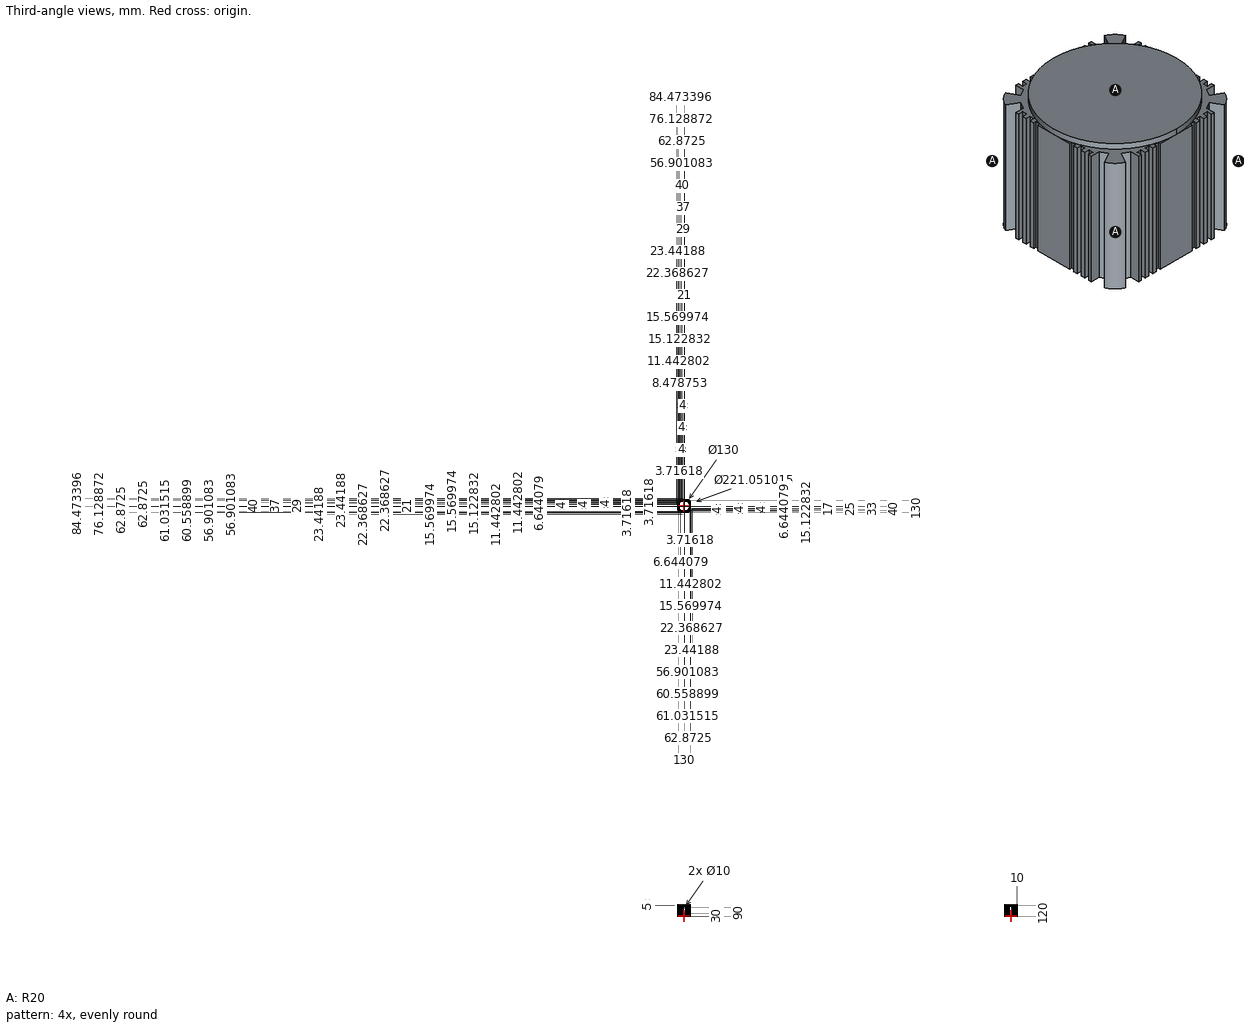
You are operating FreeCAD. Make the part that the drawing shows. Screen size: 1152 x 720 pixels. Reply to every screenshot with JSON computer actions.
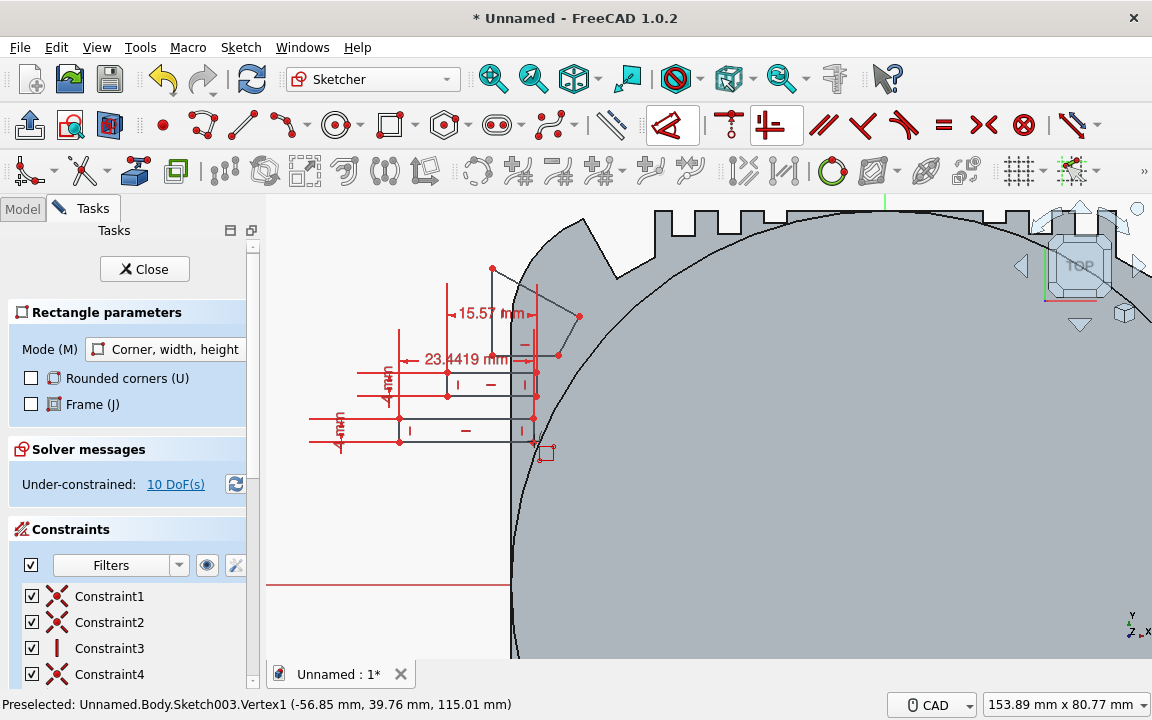
{"action": "left_click", "coordinate": [395, 464]}
{"action": "mouse_move", "coordinate": [523, 487]}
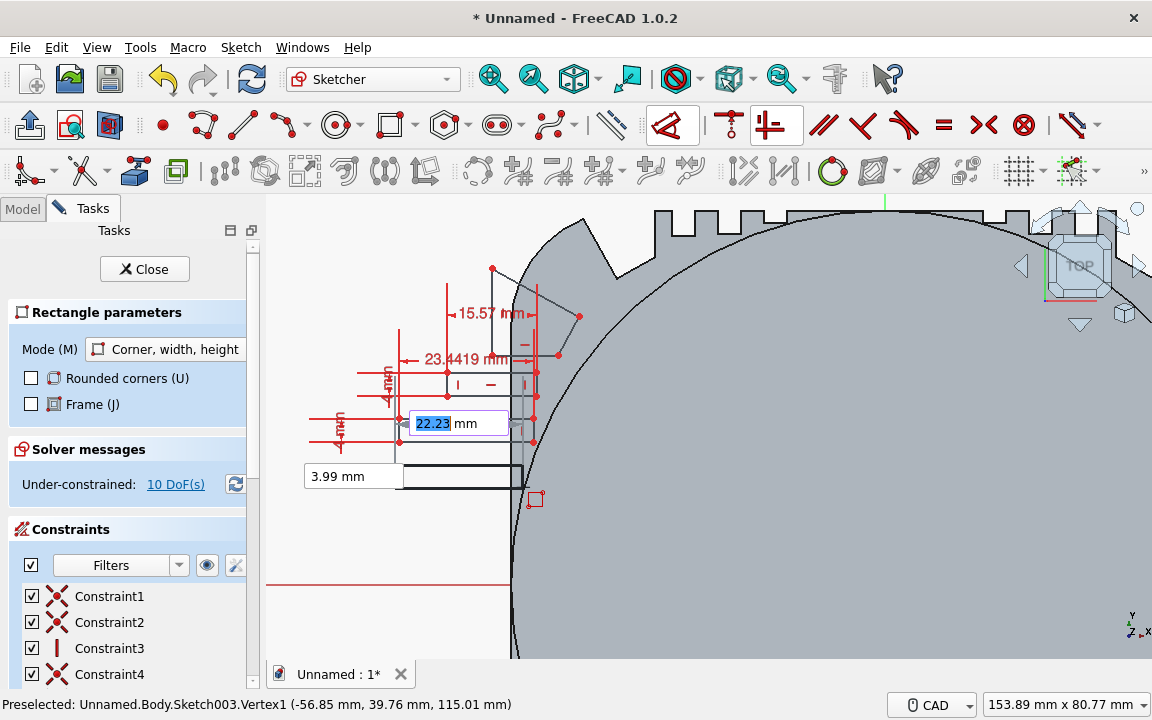
{"action": "type", "text": "22.368627"}
{"action": "key", "text": "Tab"}
{"action": "type", "text": "4"}
{"action": "key", "text": "Return"}
{"action": "key", "text": "Escape"}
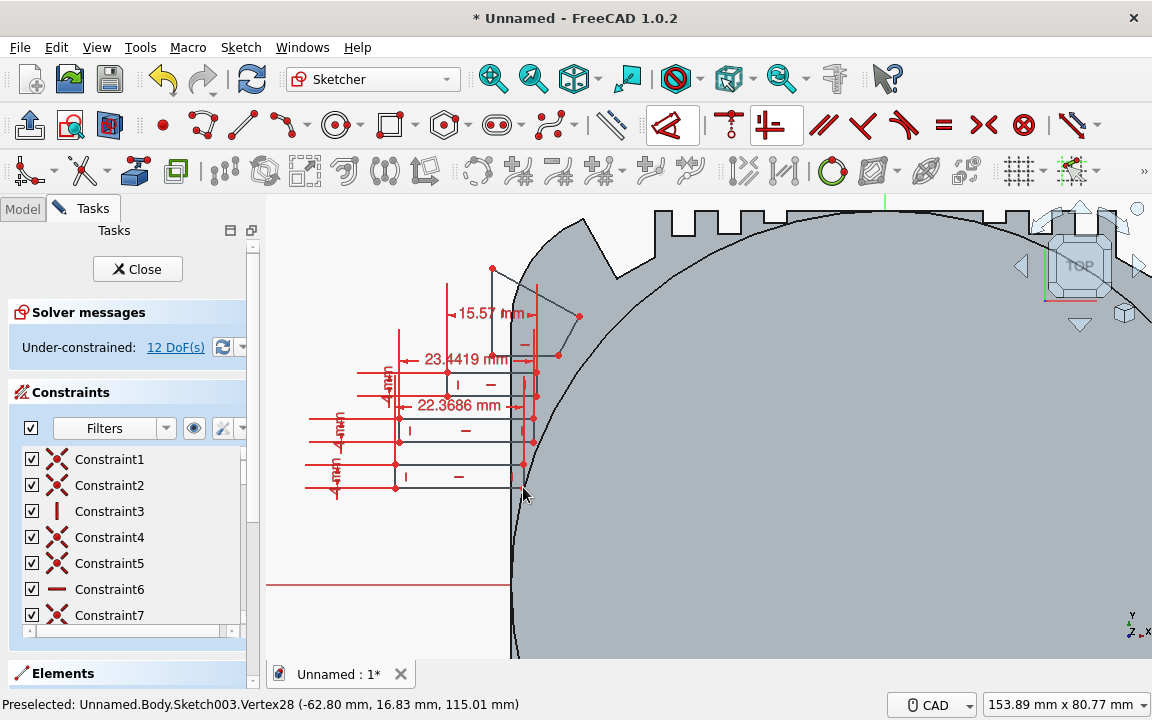
{"action": "left_click", "coordinate": [558, 356]}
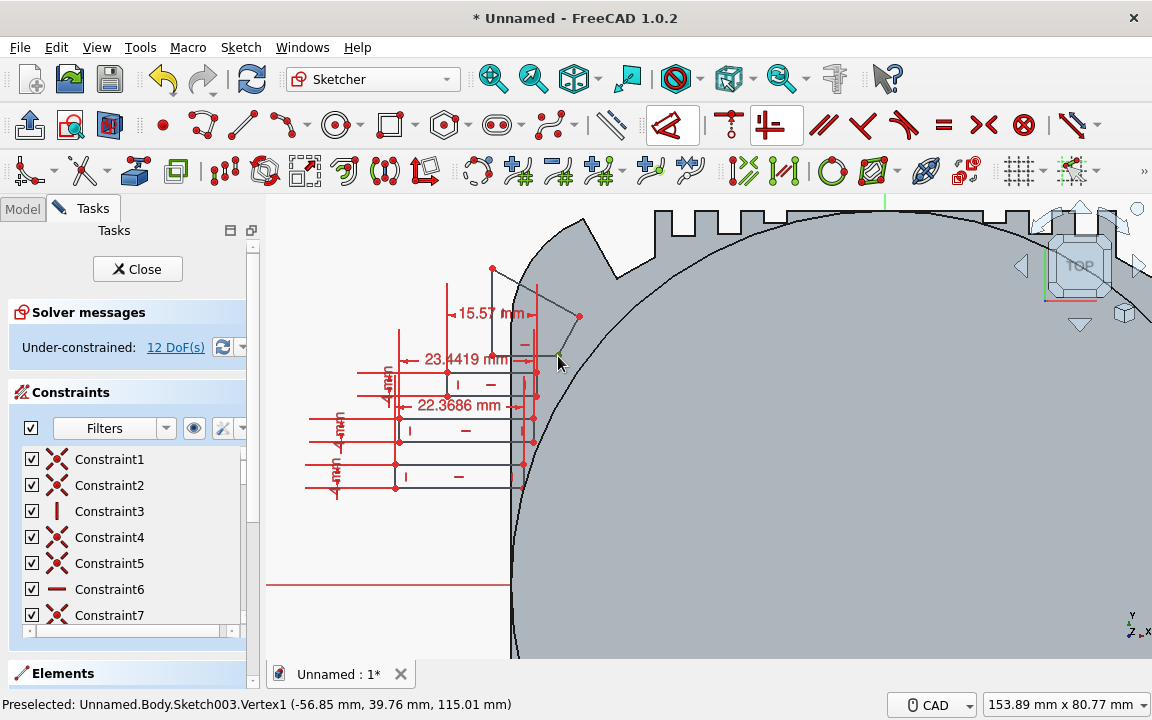
{"action": "key", "text": "i"}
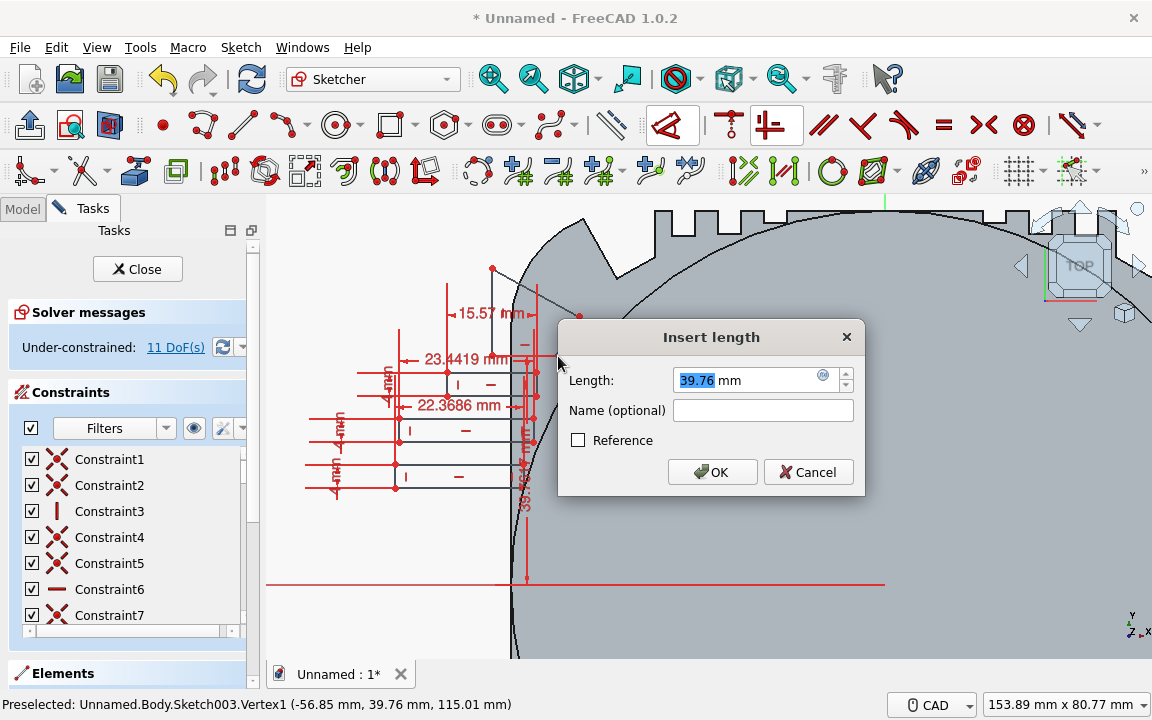
{"action": "type", "text": "40"}
{"action": "key", "text": "Return"}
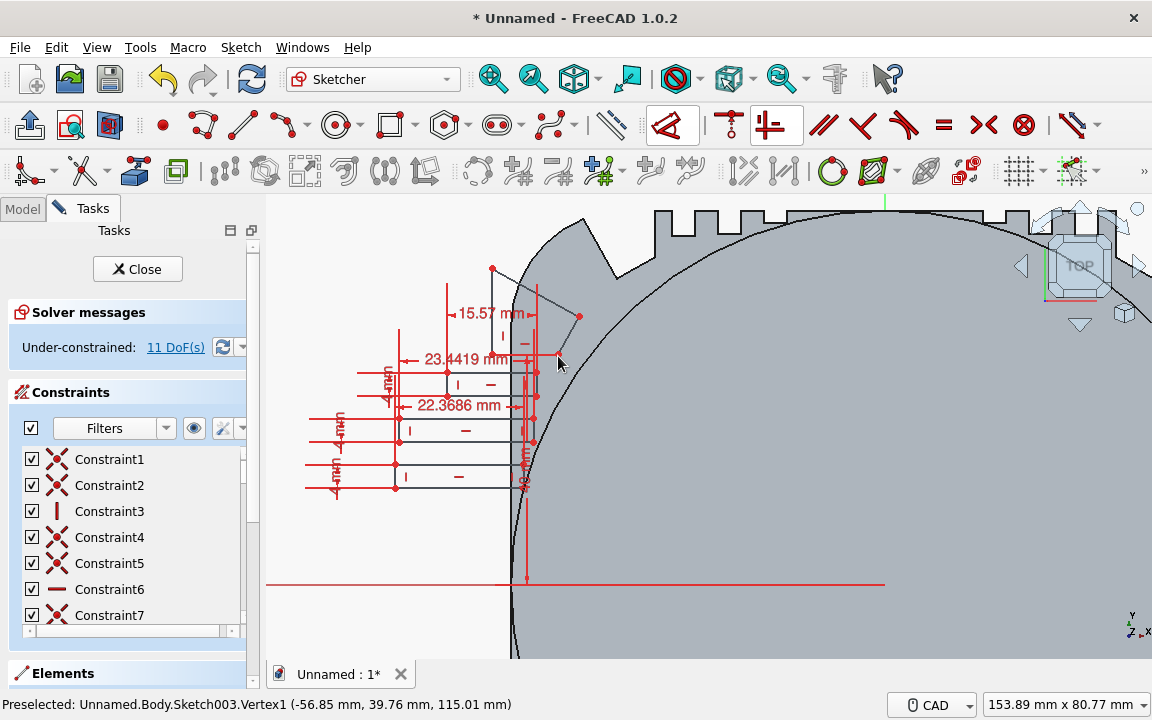
{"action": "left_click", "coordinate": [447, 373]}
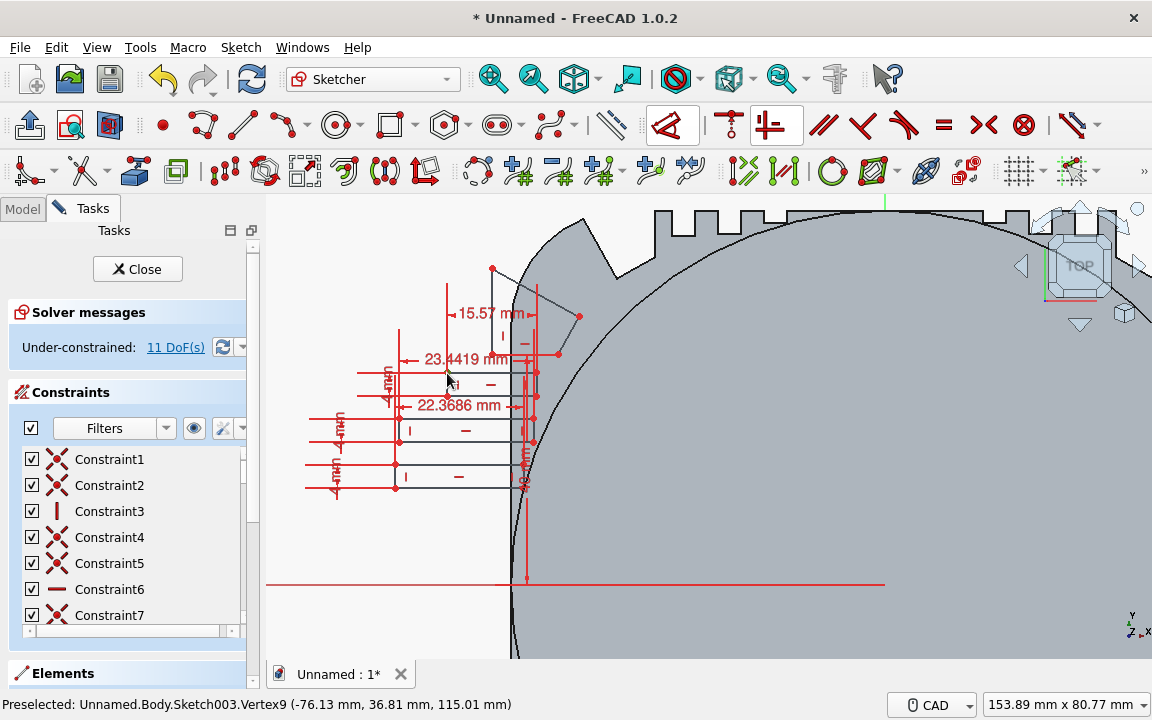
{"action": "left_click", "coordinate": [694, 126]}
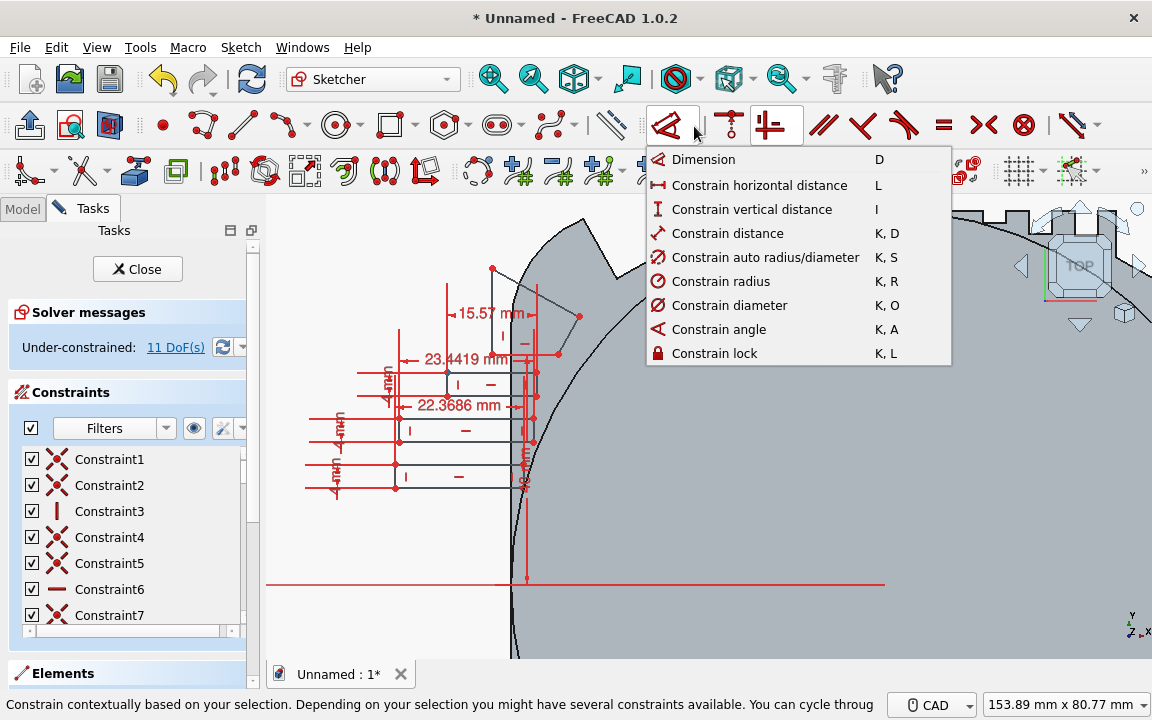
{"action": "left_click", "coordinate": [799, 209]}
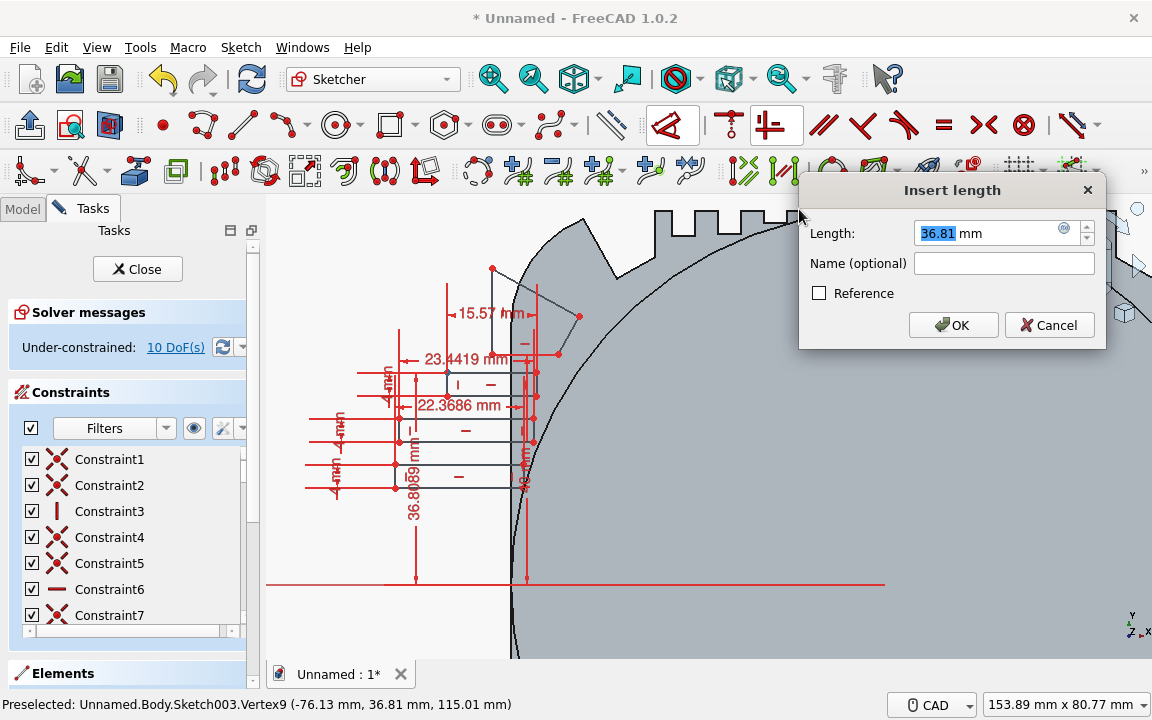
{"action": "type", "text": "37"}
{"action": "key", "text": "Return"}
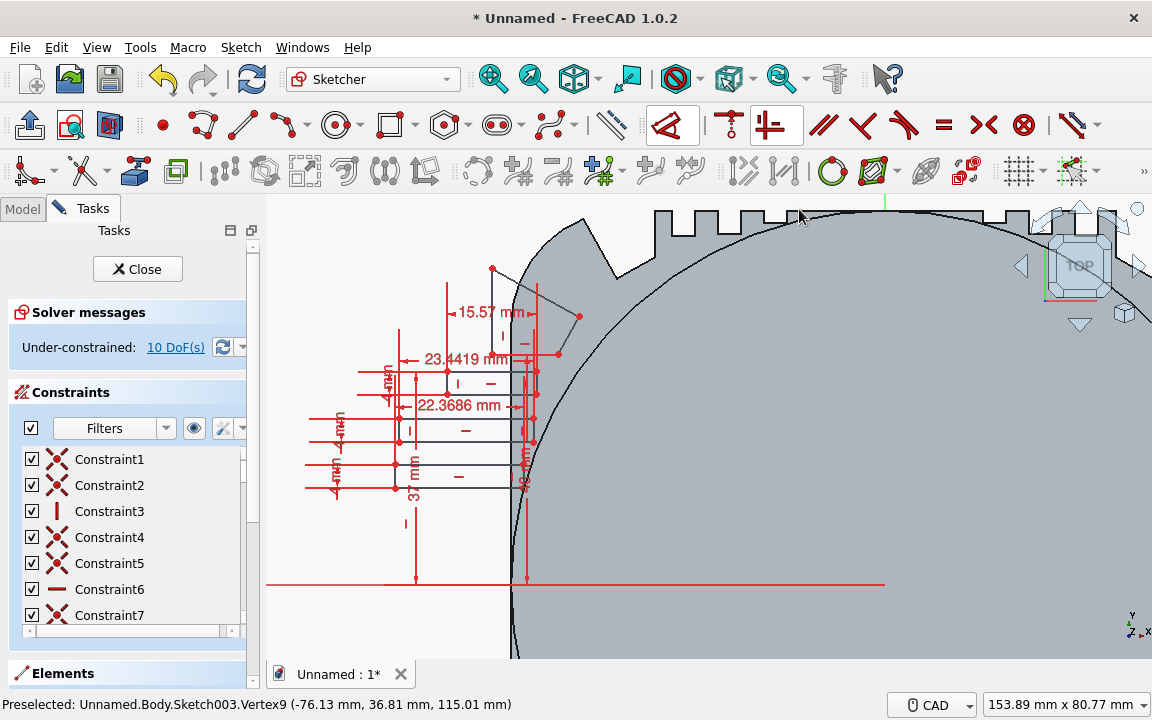
{"action": "left_click", "coordinate": [399, 419]}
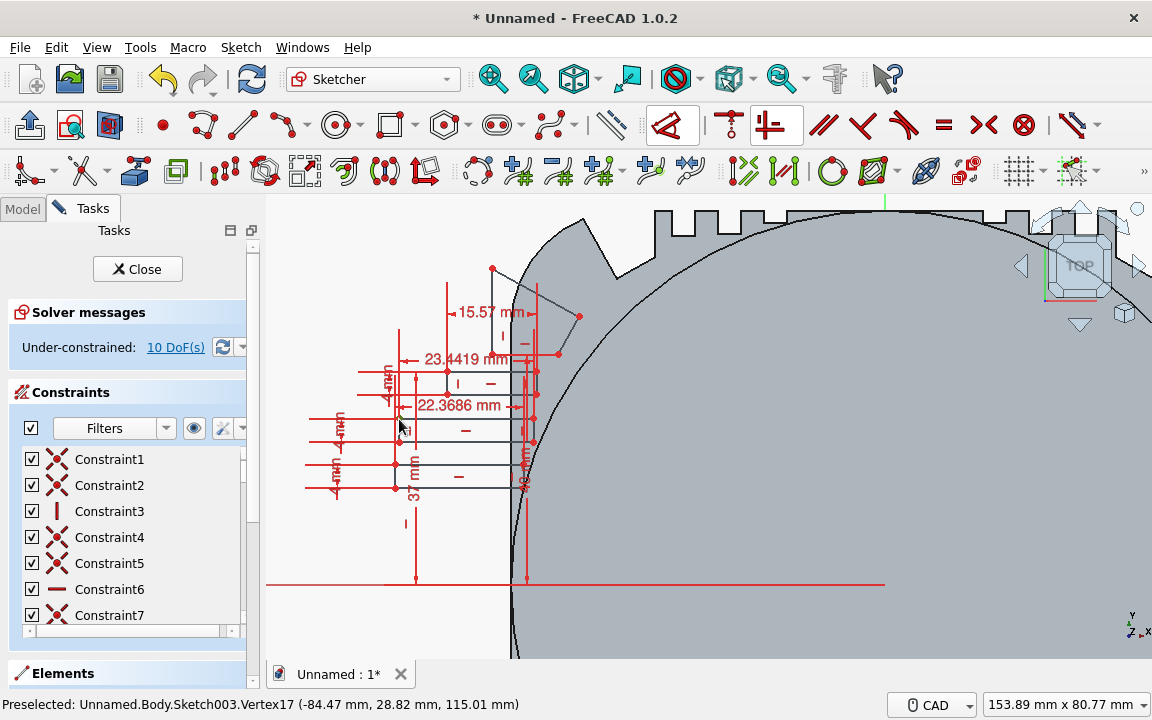
{"action": "key", "text": "i"}